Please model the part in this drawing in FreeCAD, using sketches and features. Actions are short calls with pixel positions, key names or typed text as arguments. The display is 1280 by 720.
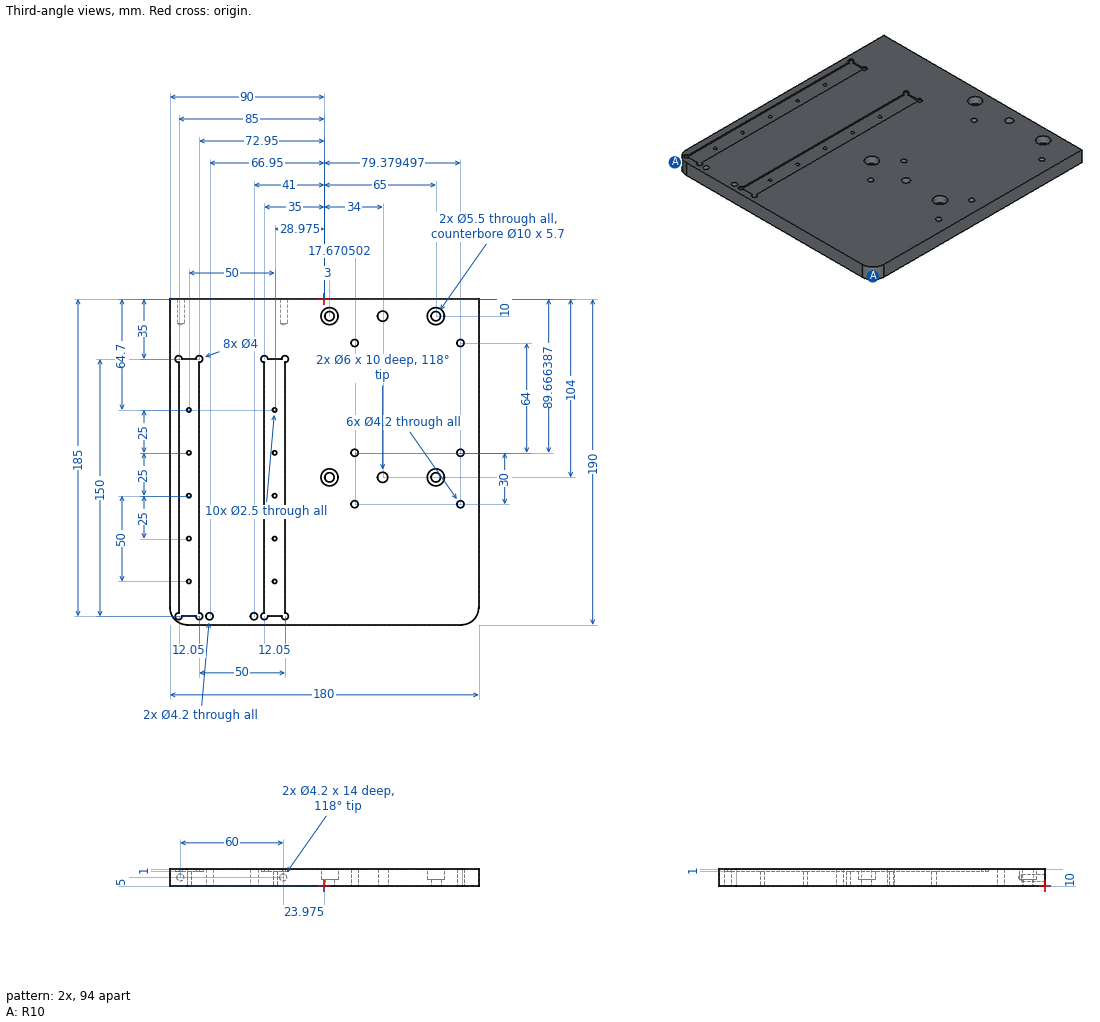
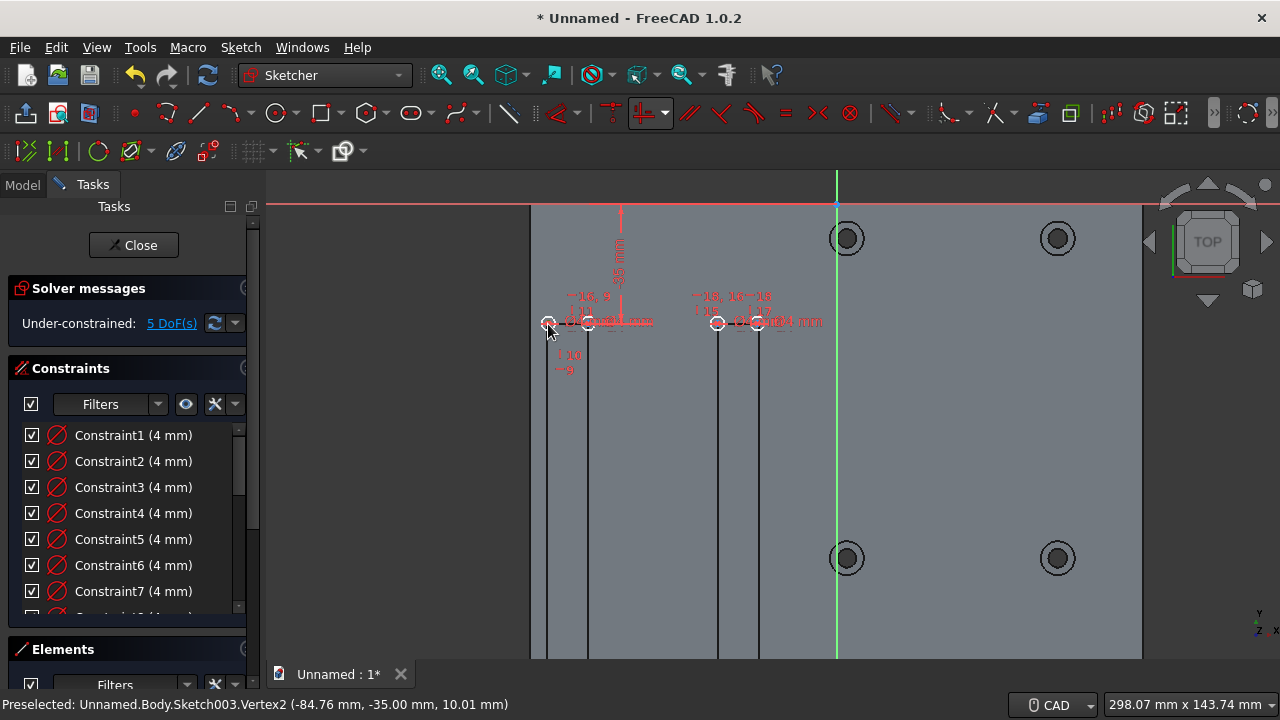
key(l)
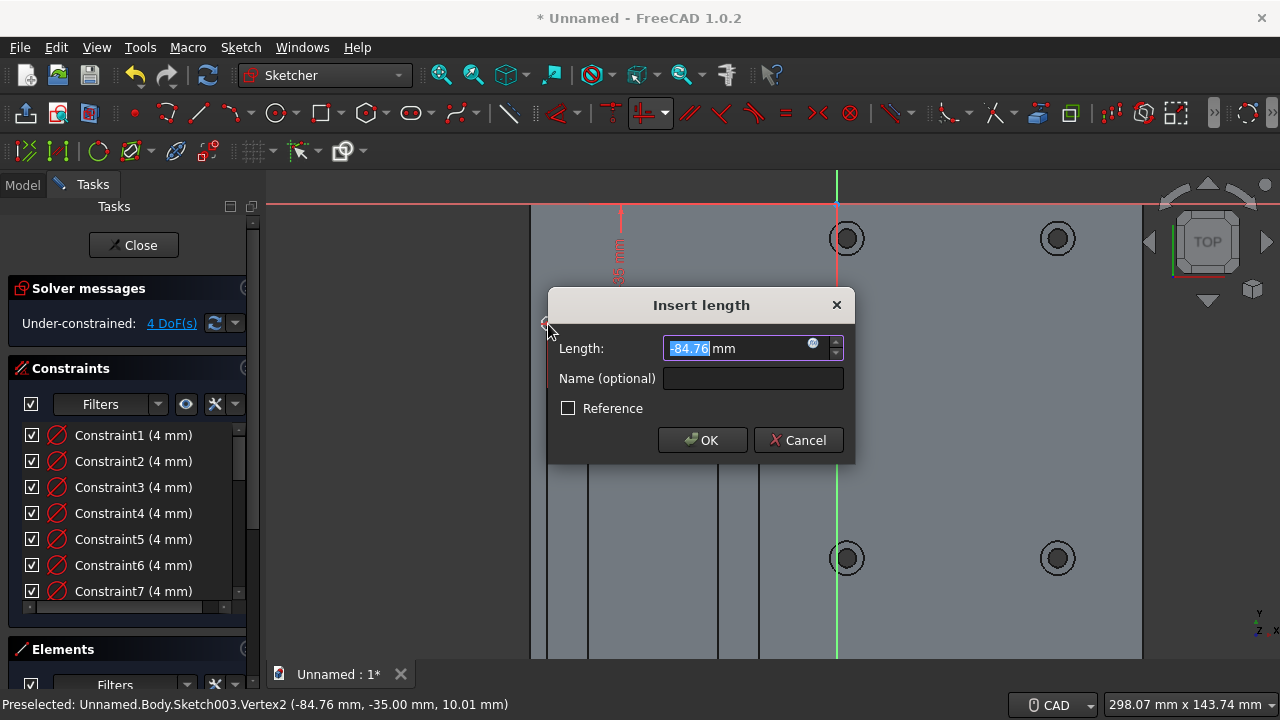
text(-85)
key(Return)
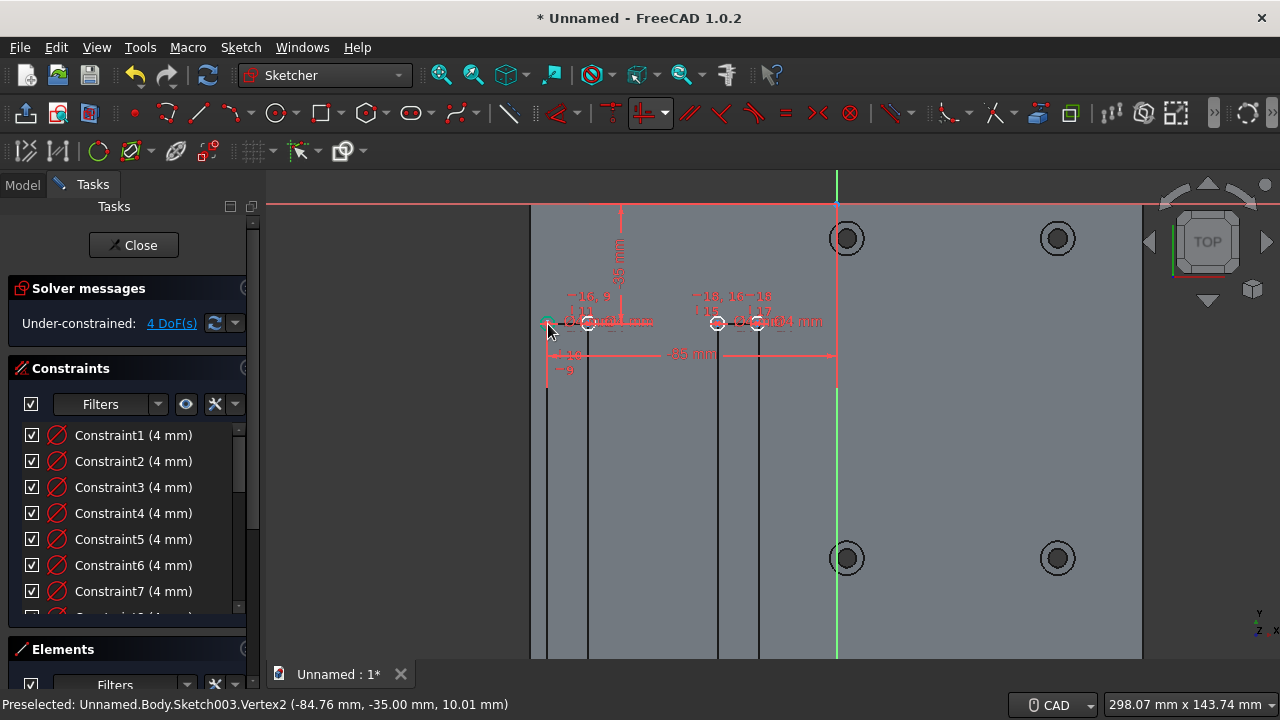
scroll(717, 326, down, 4)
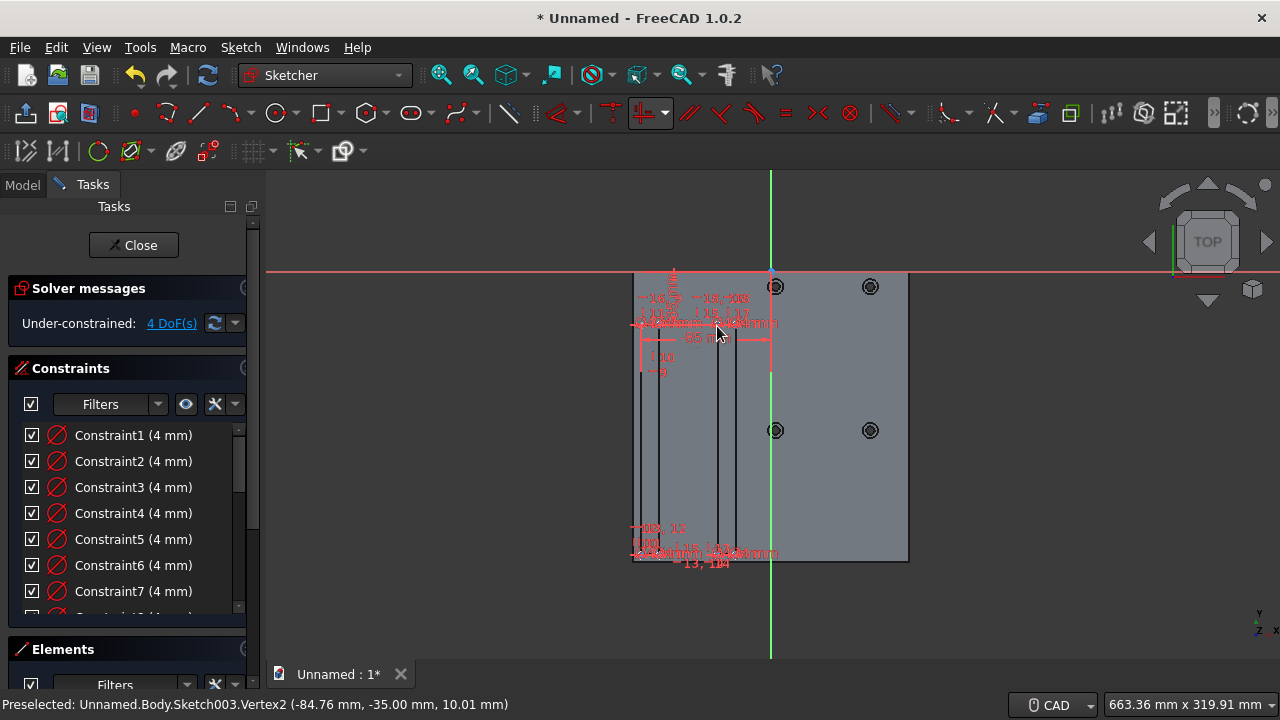
click(717, 555)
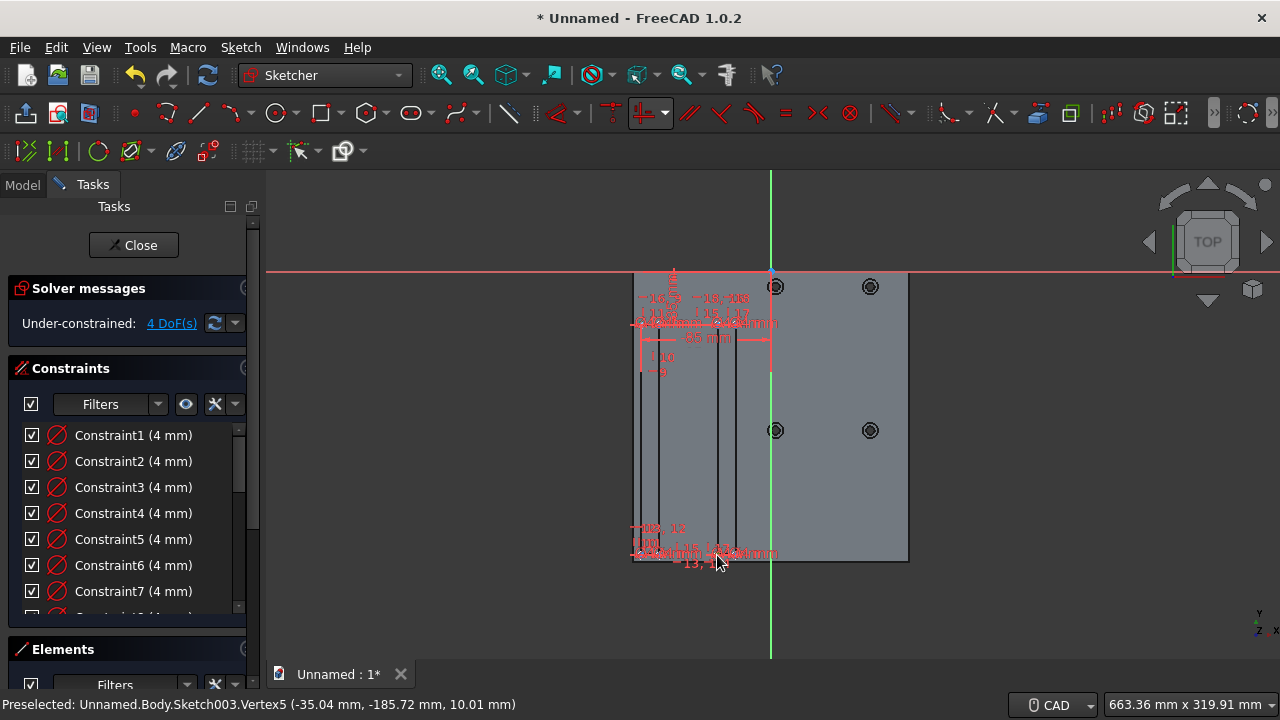
key(l)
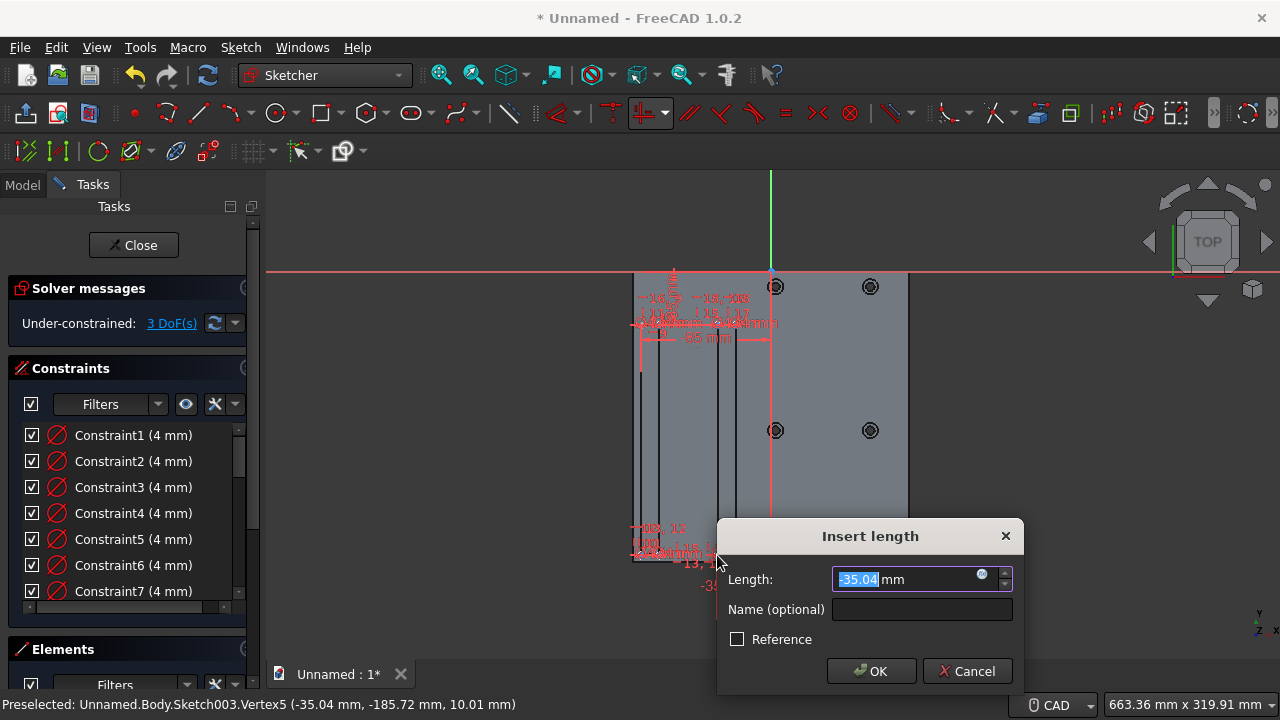
text(-35)
key(Return)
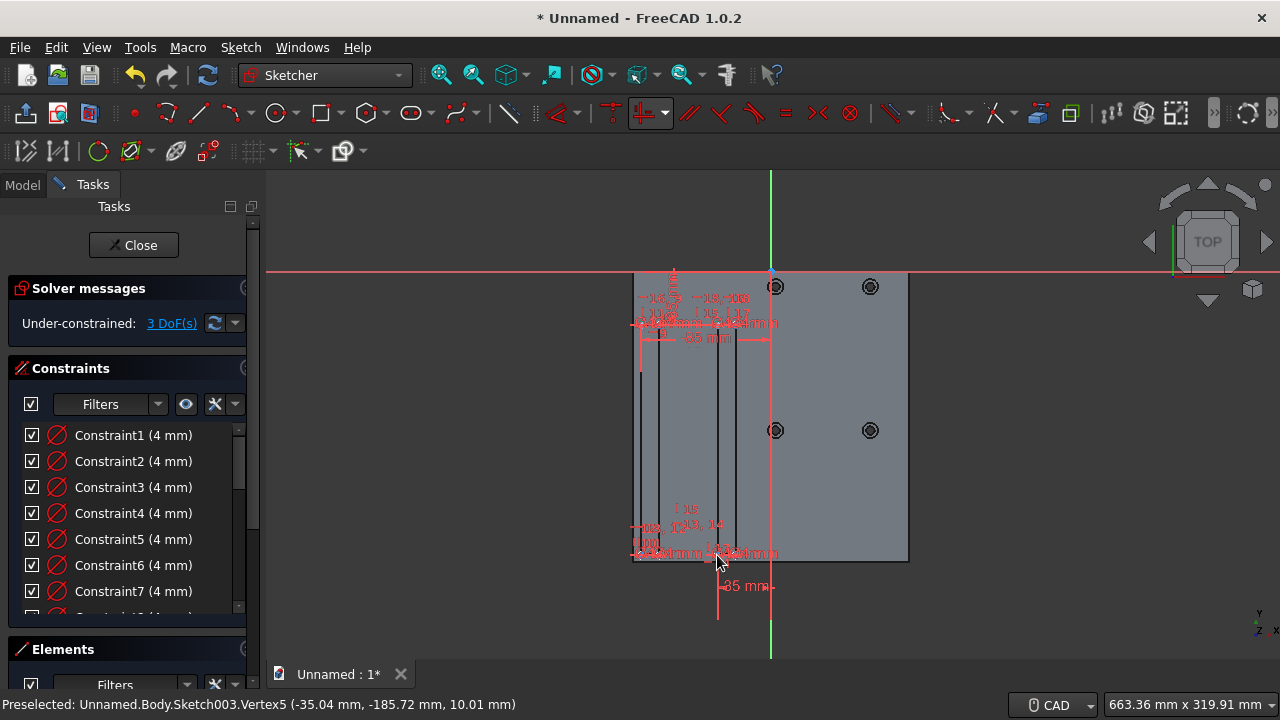
click(641, 555)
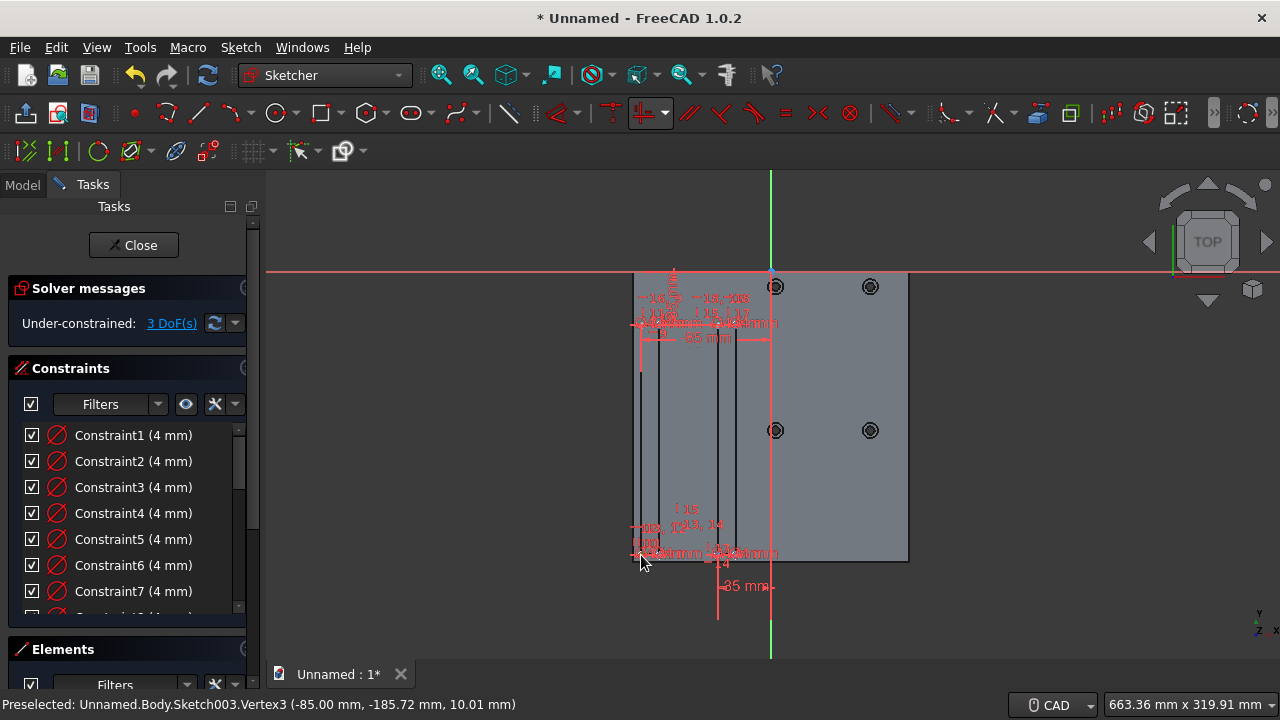
click(580, 114)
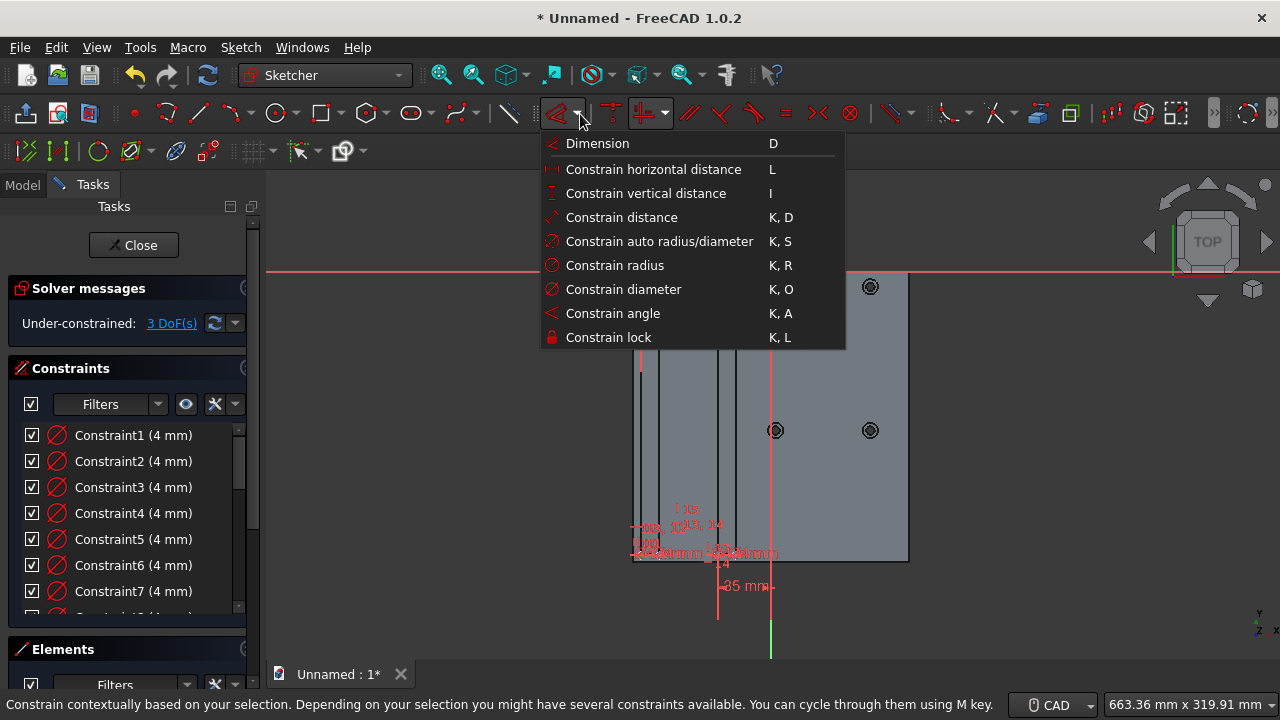
click(693, 193)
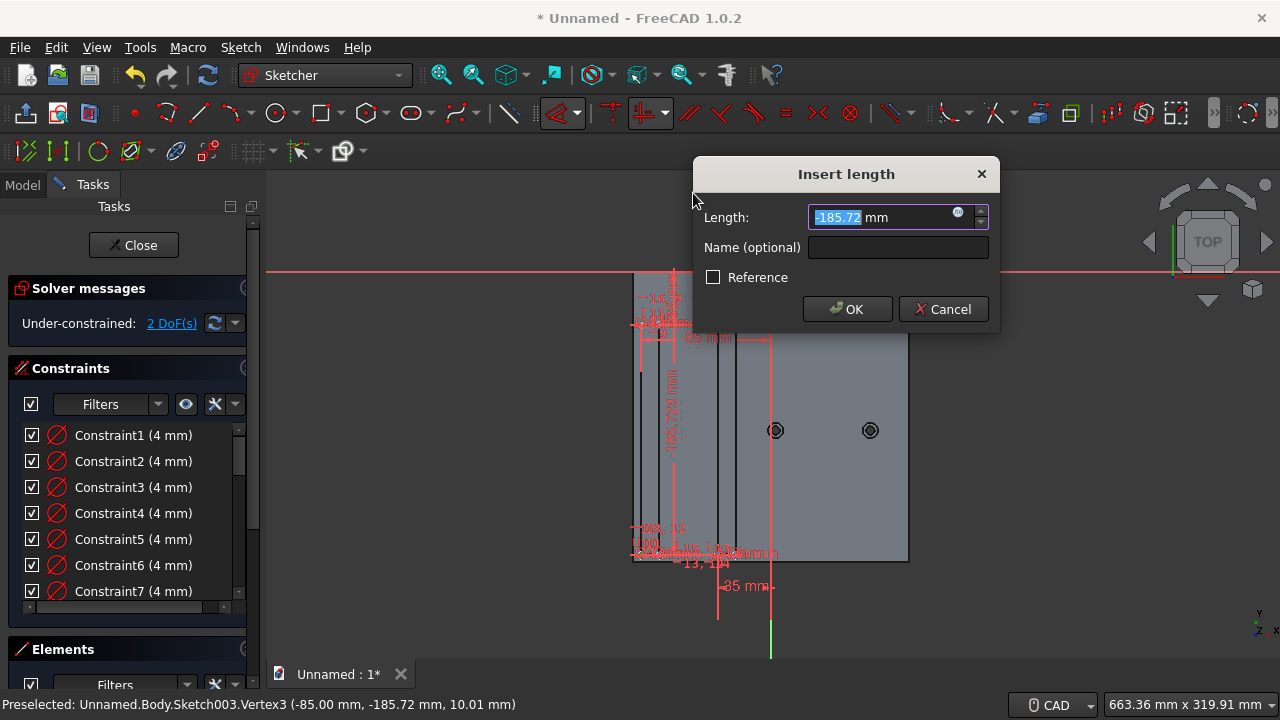
text(-185)
key(Return)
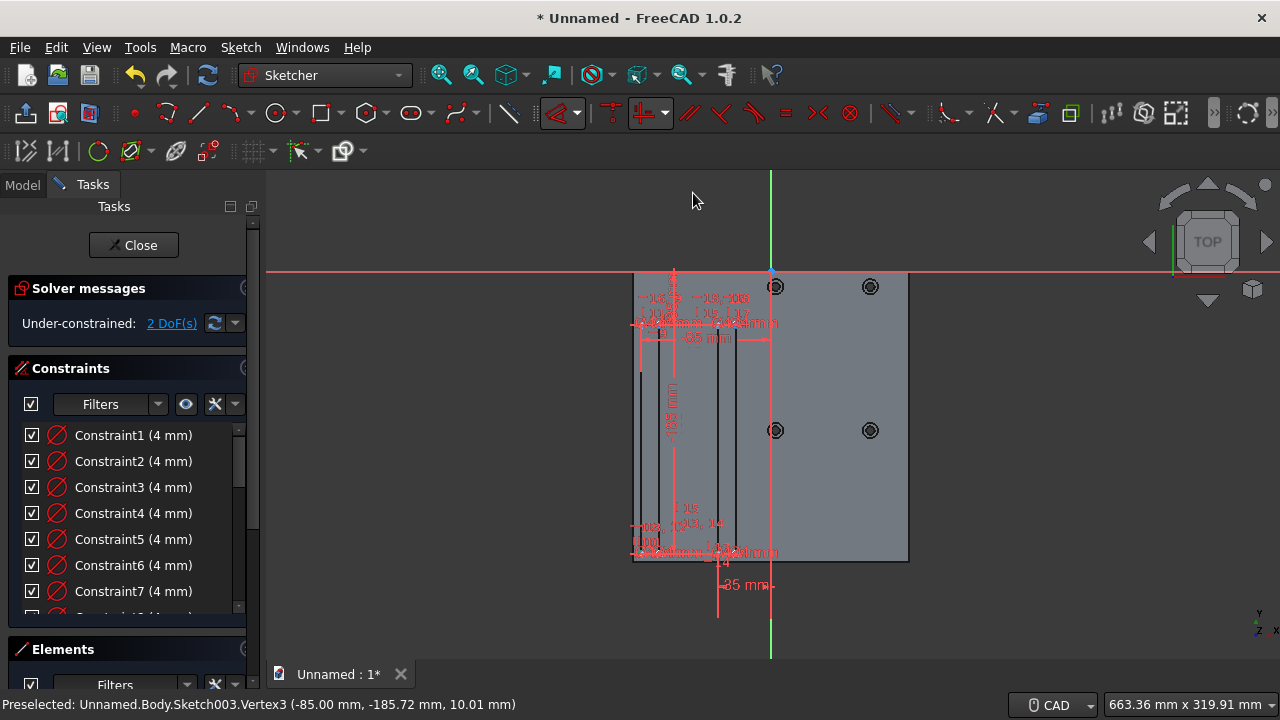
click(659, 554)